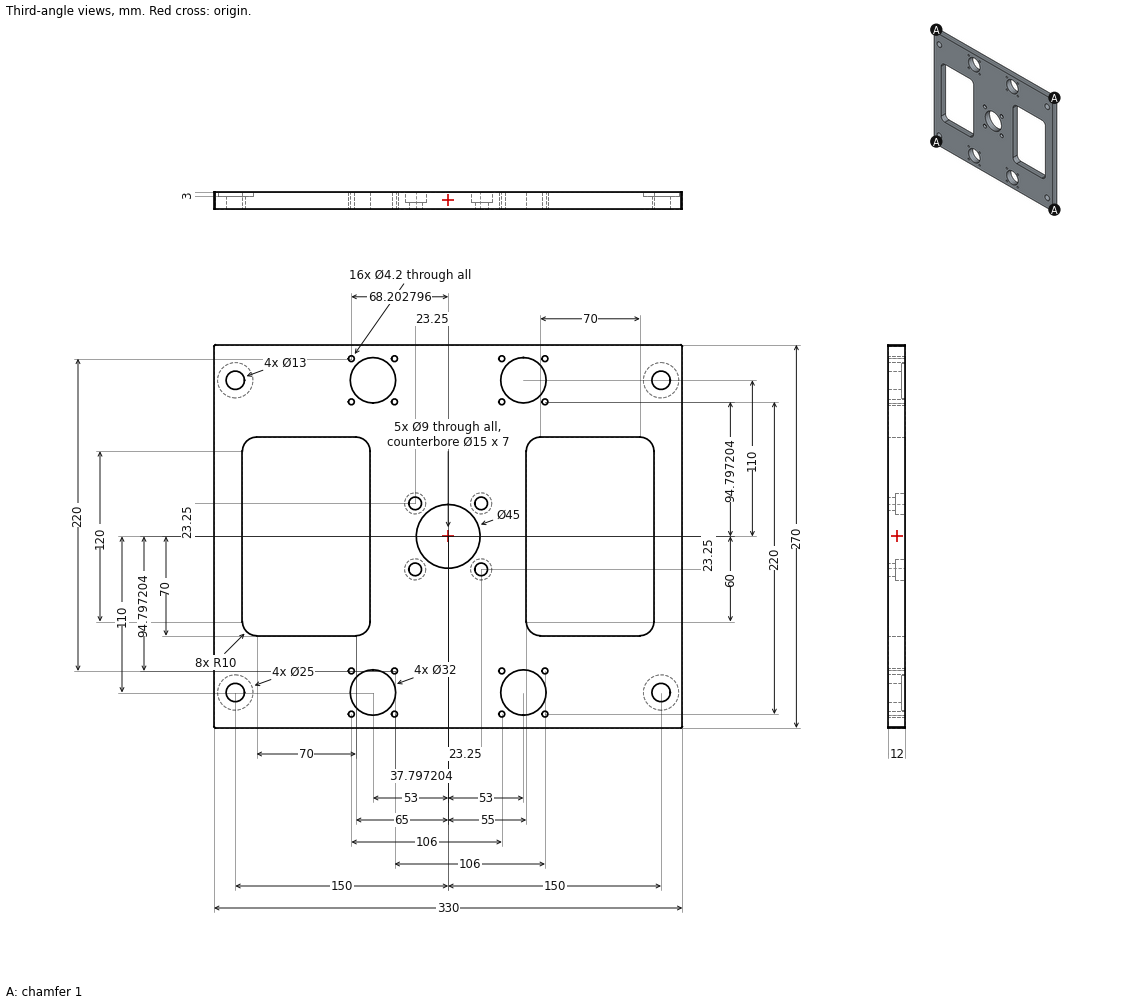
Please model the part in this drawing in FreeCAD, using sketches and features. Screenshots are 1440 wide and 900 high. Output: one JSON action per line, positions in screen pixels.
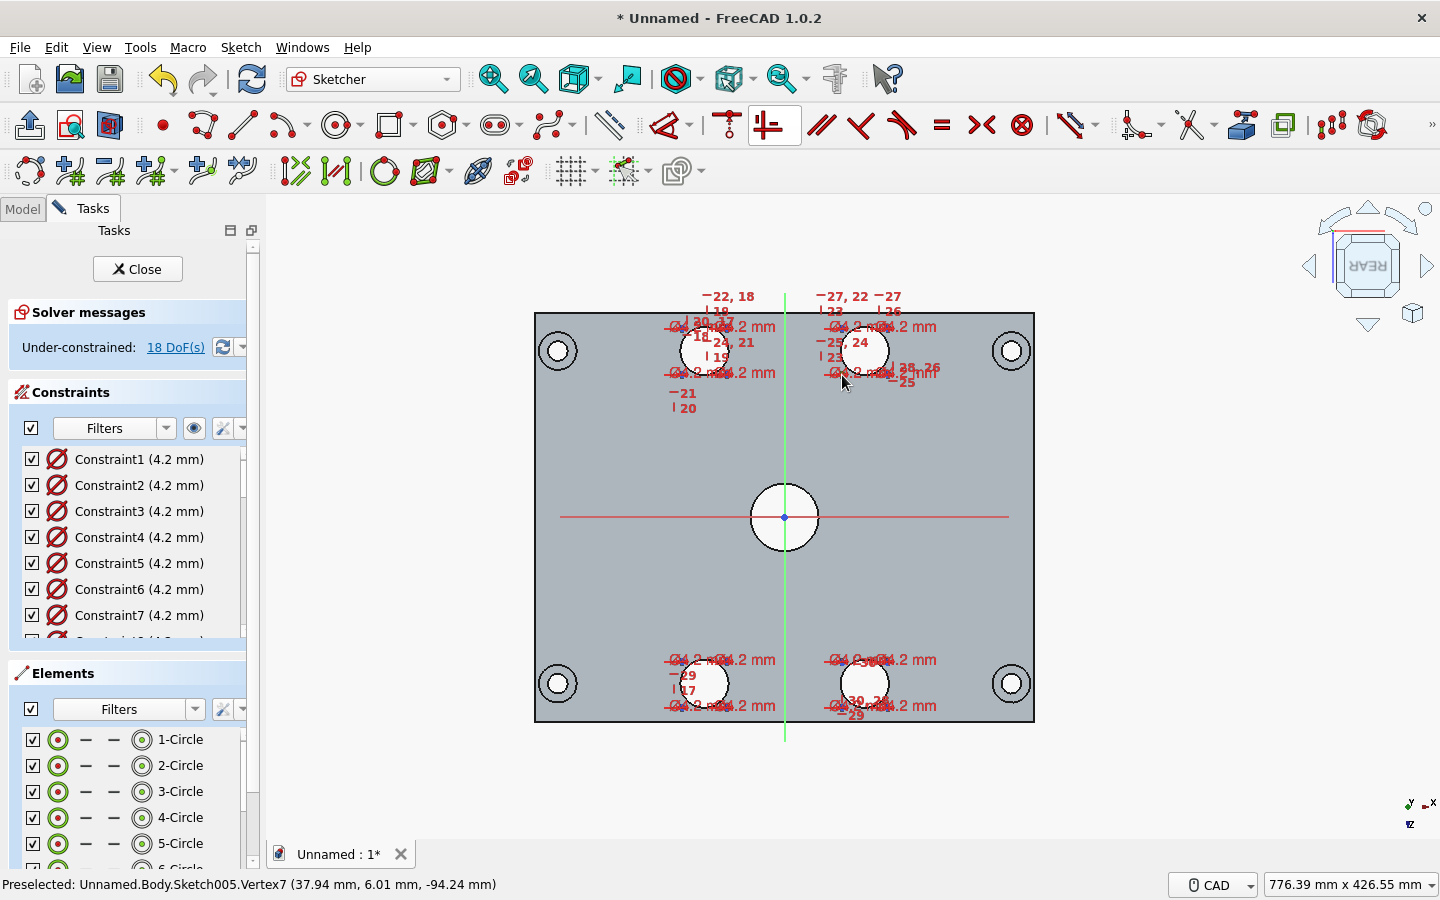
{"action": "left_click", "coordinate": [842, 662]}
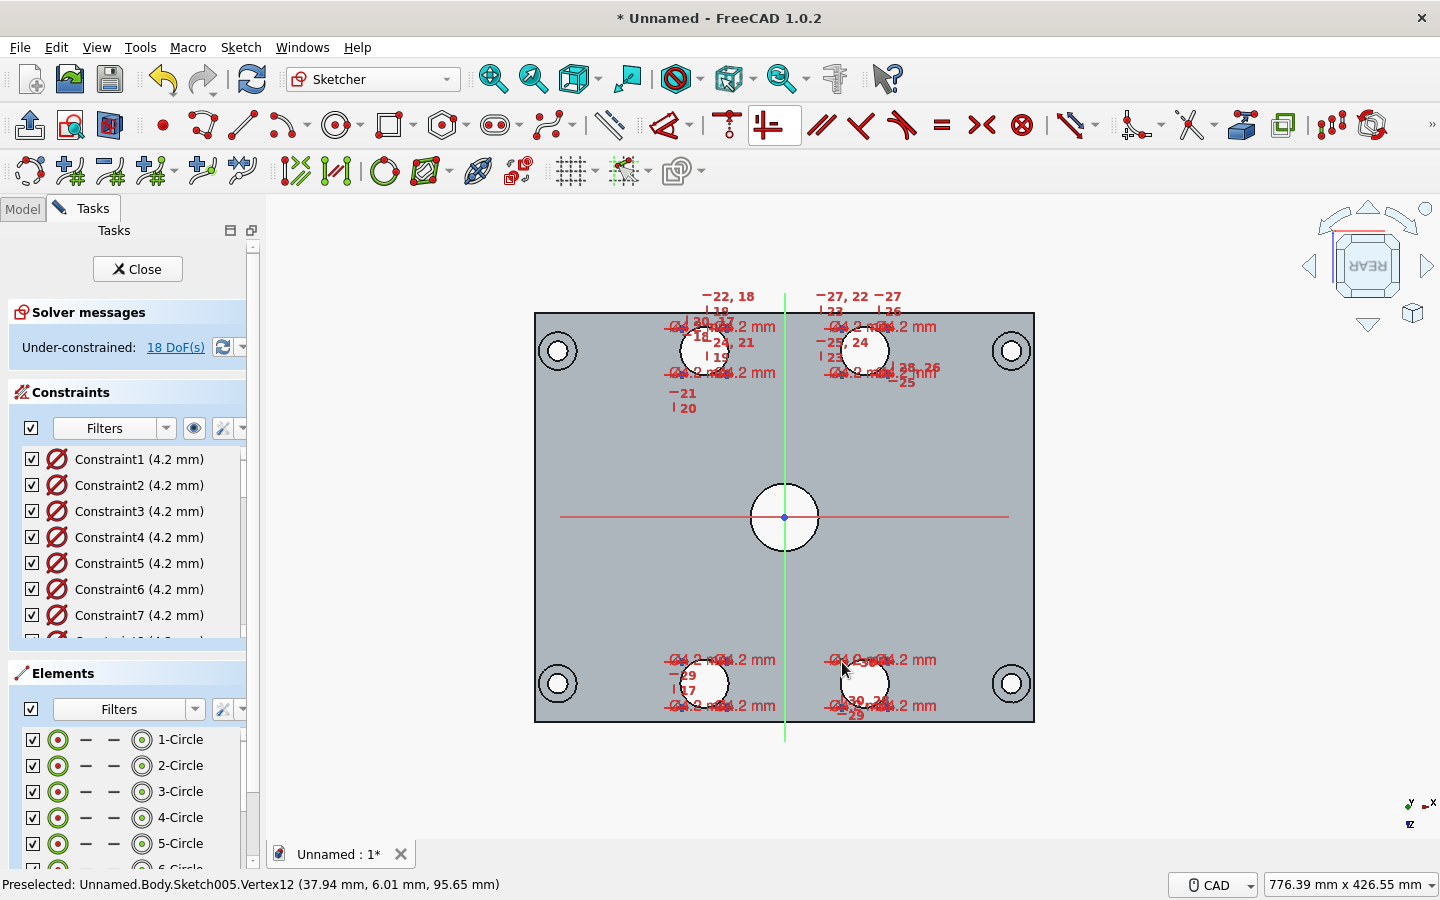
{"action": "left_click", "coordinate": [796, 126]}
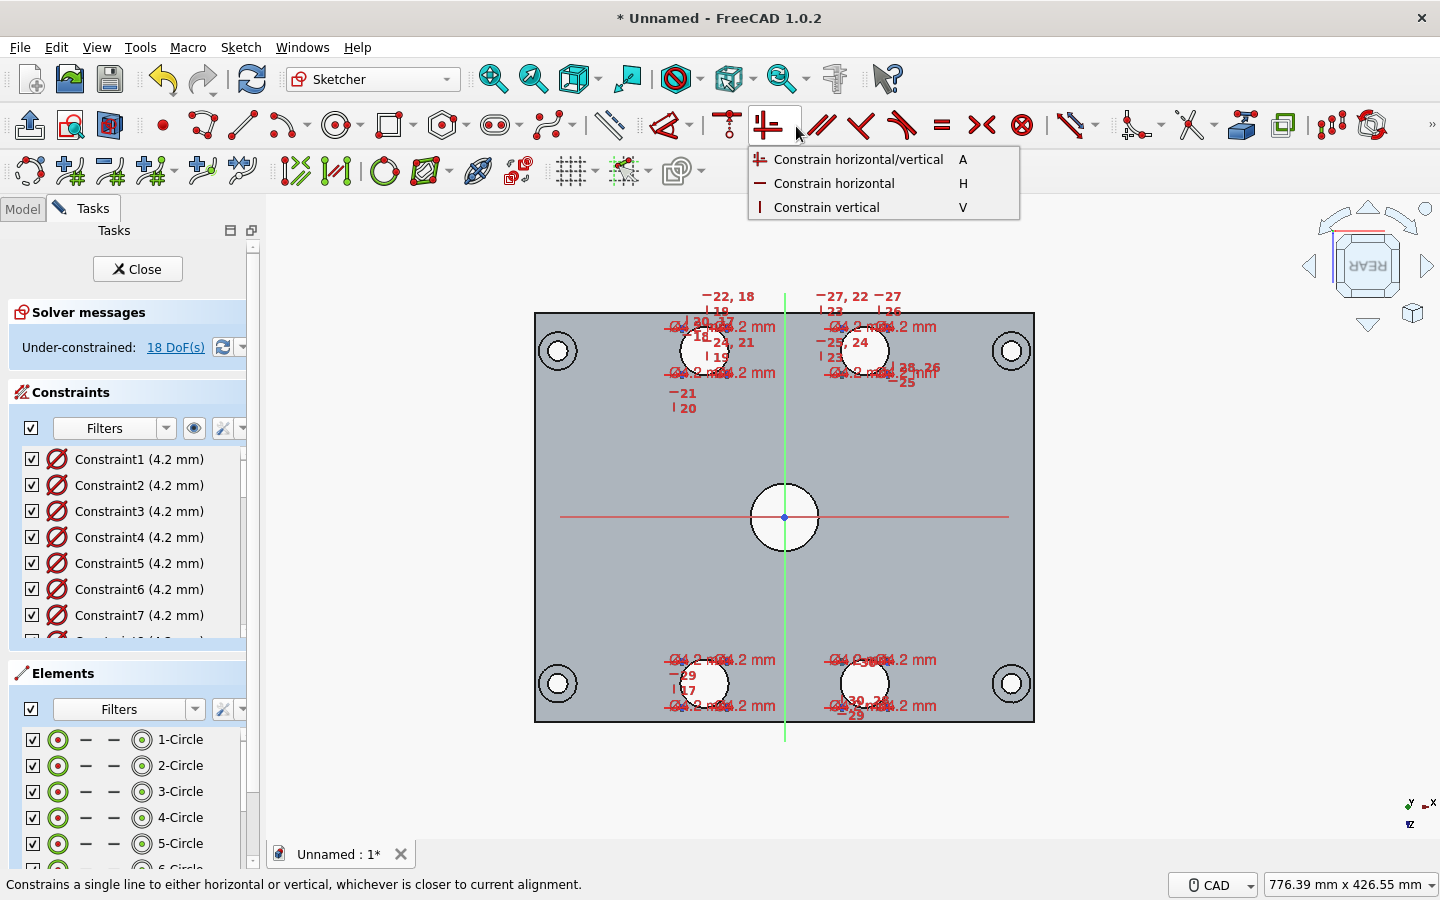
{"action": "left_click", "coordinate": [884, 207]}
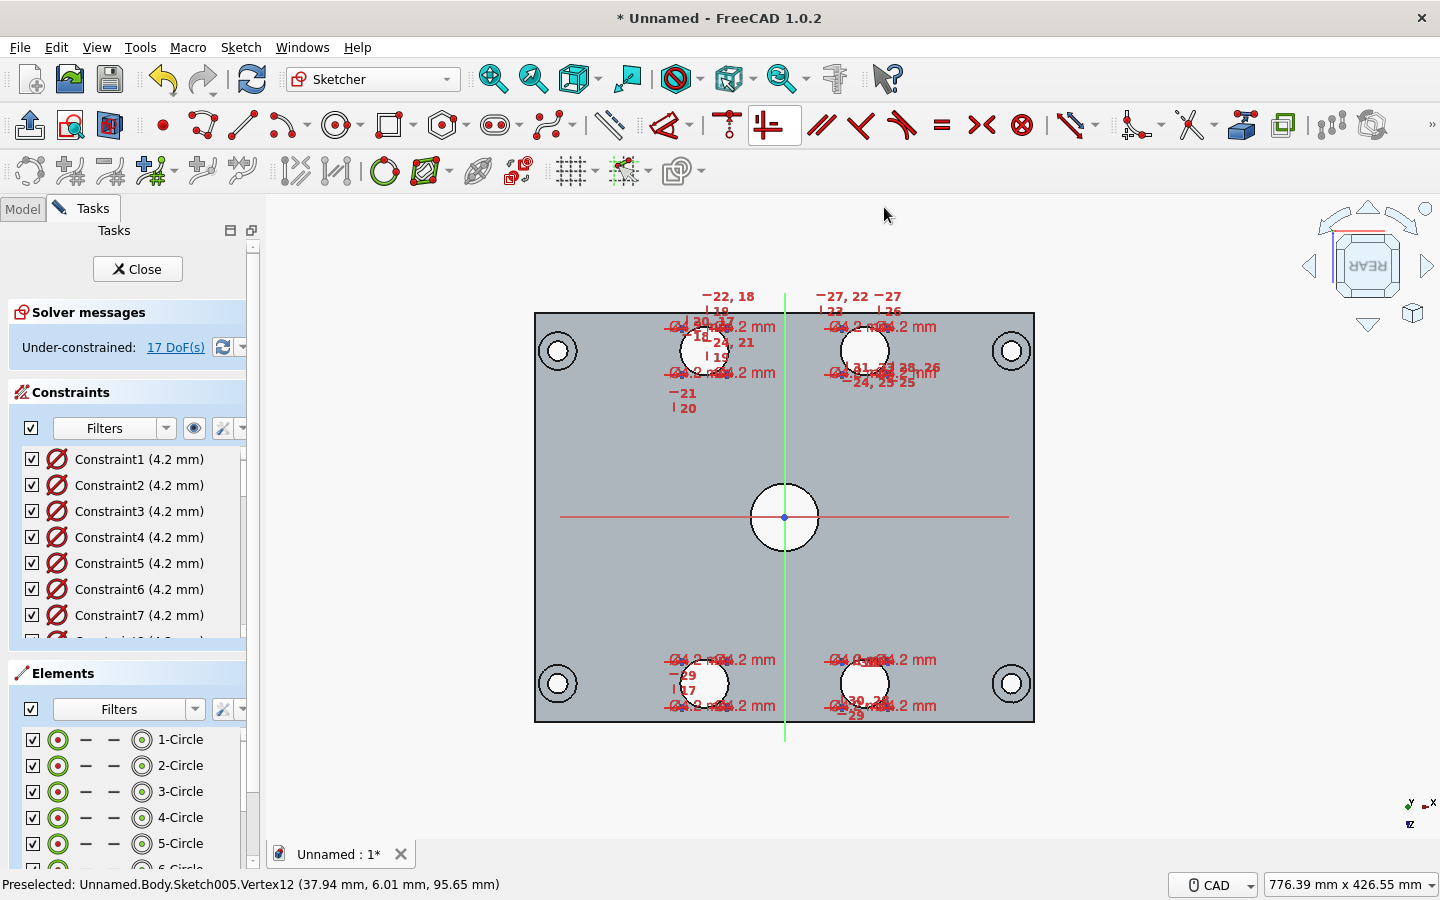
{"action": "left_click", "coordinate": [888, 662]}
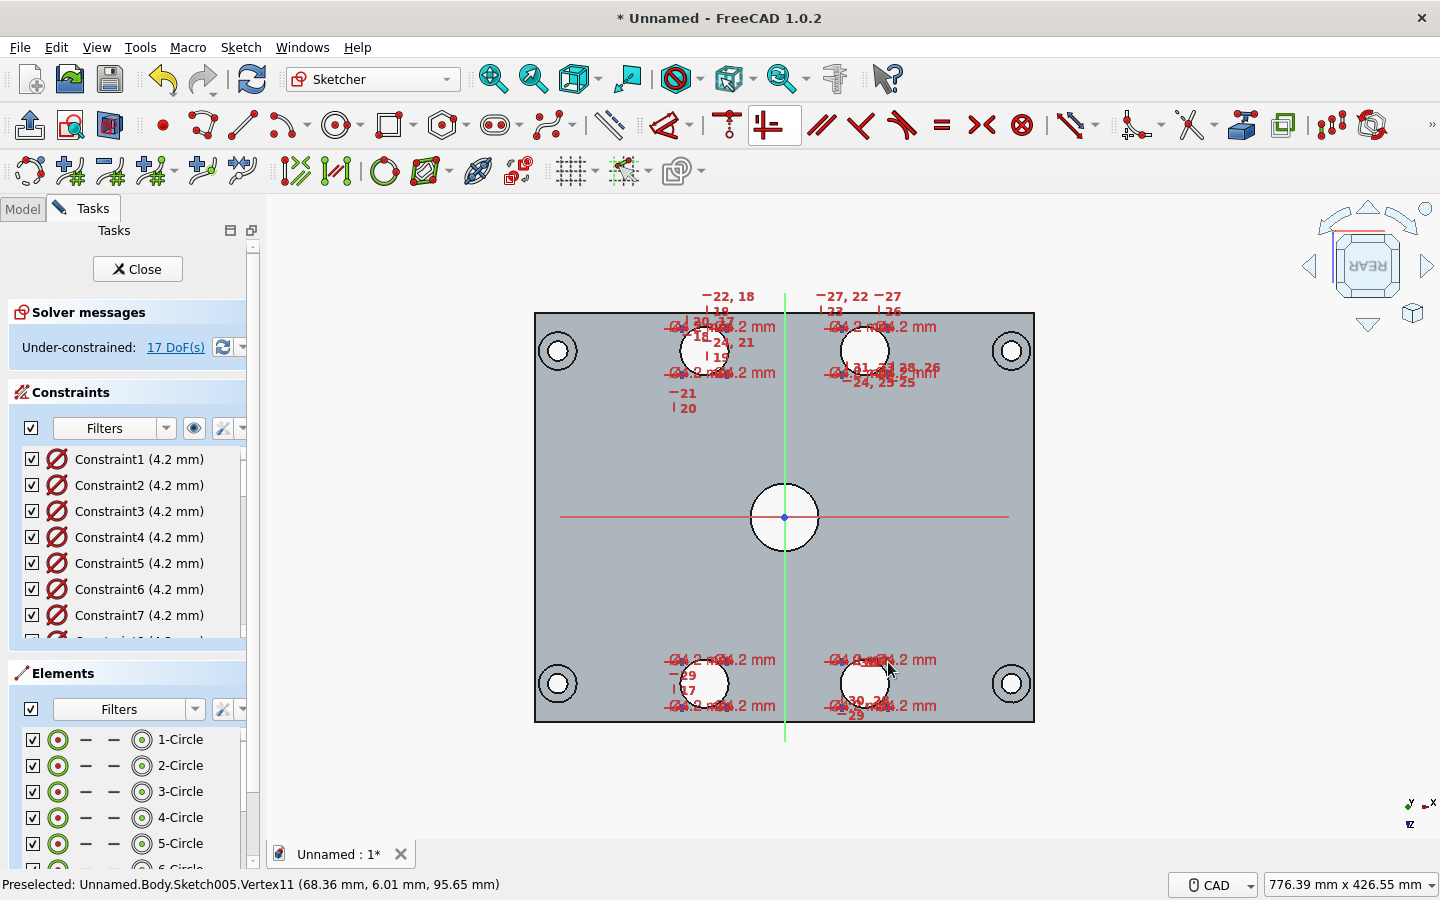
{"action": "left_click", "coordinate": [842, 662]}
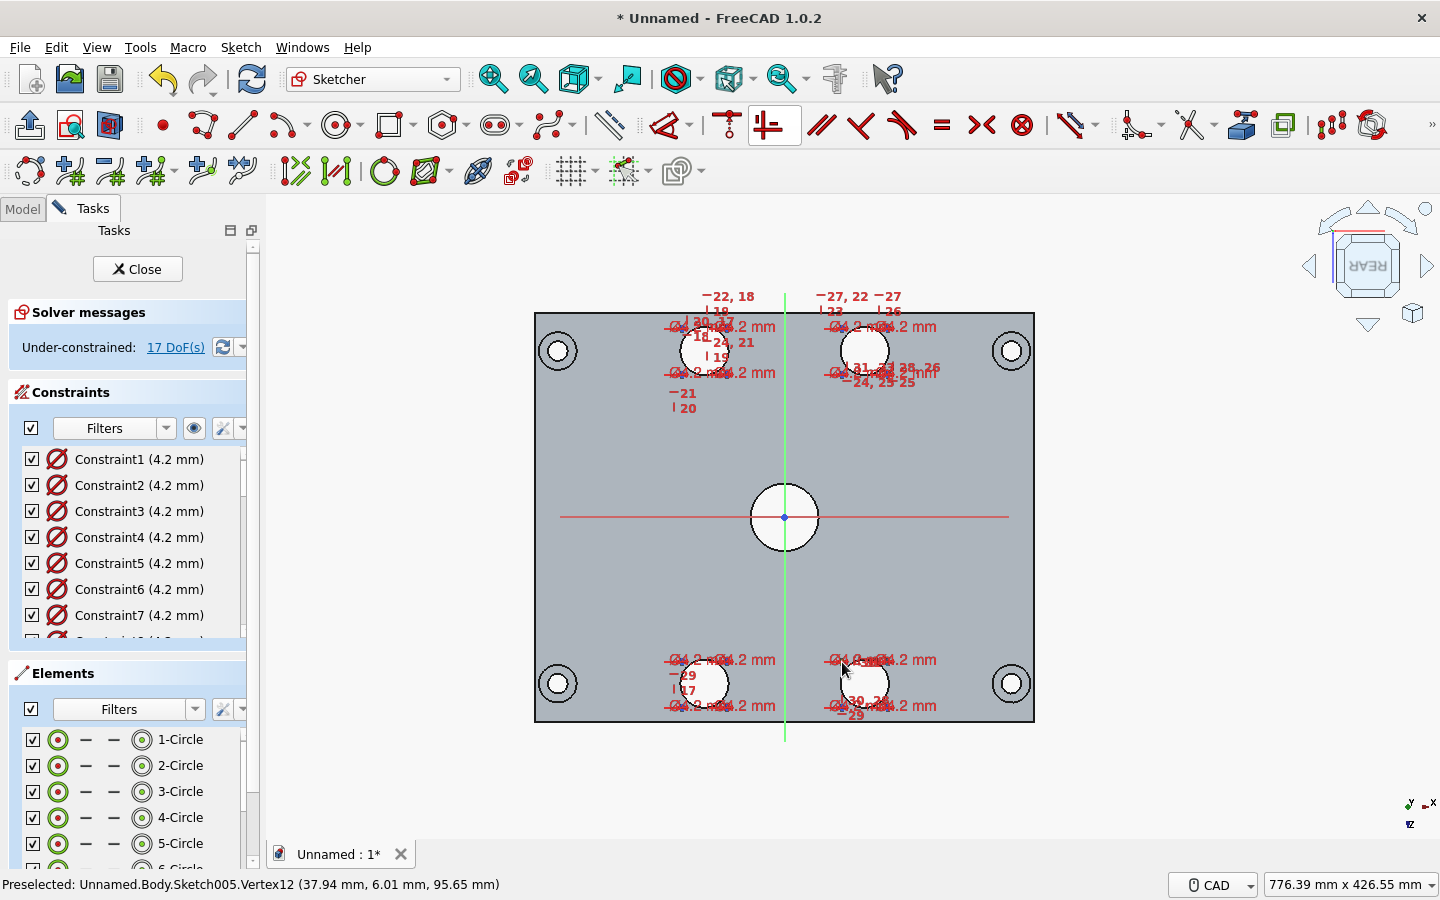
{"action": "left_click", "coordinate": [796, 126]}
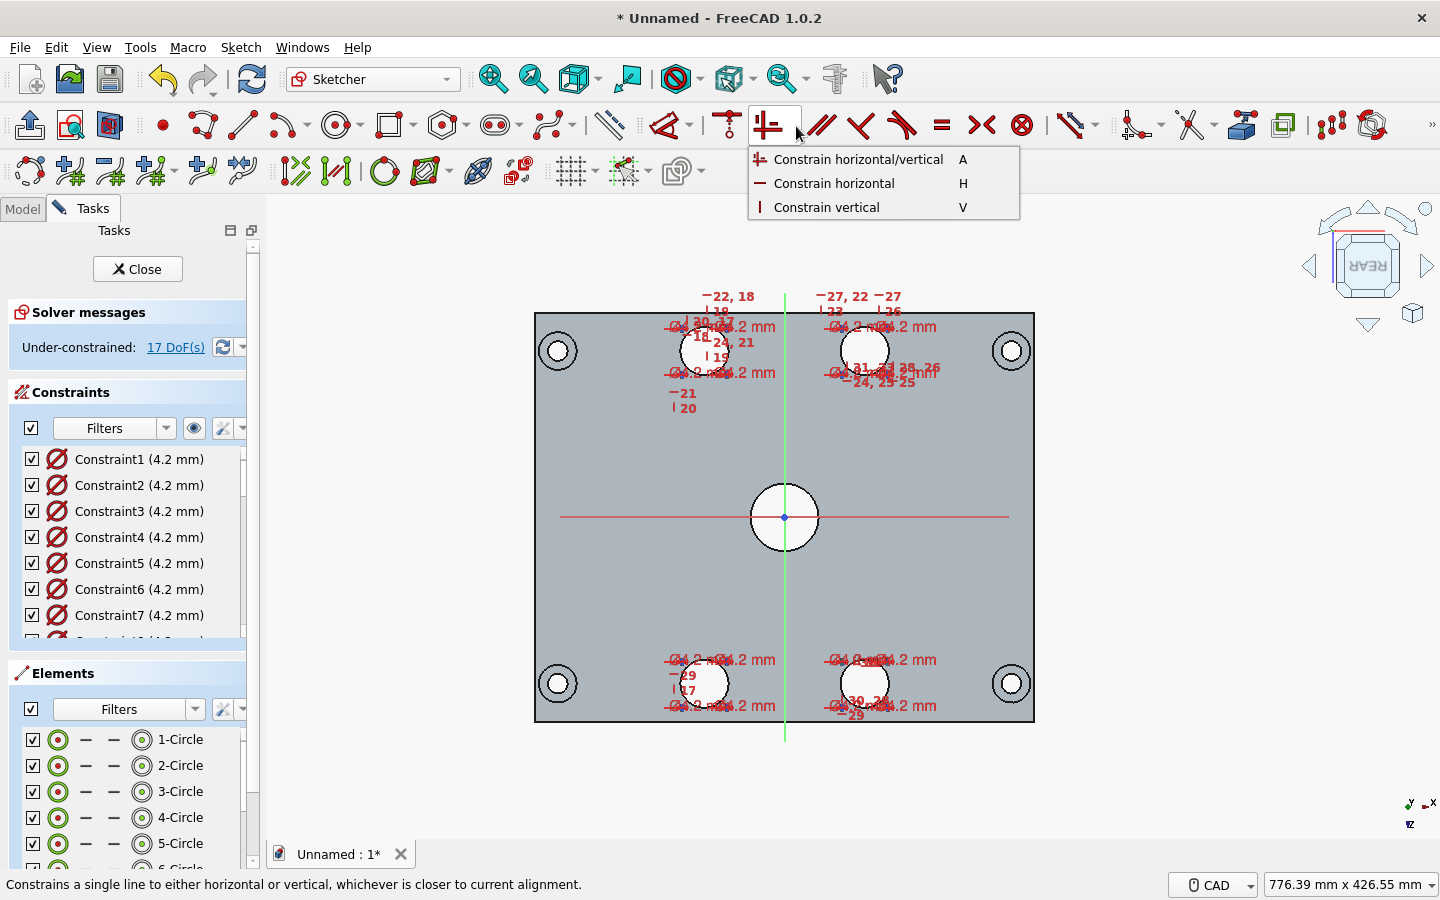
{"action": "left_click", "coordinate": [884, 183]}